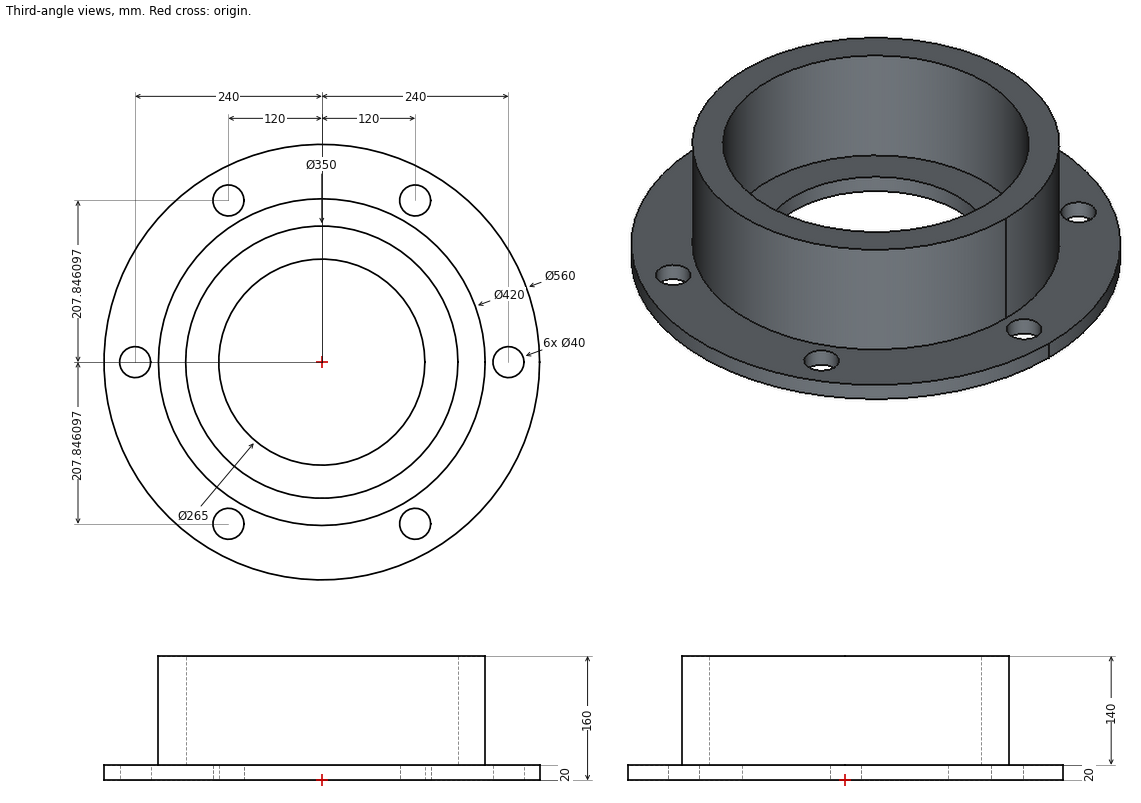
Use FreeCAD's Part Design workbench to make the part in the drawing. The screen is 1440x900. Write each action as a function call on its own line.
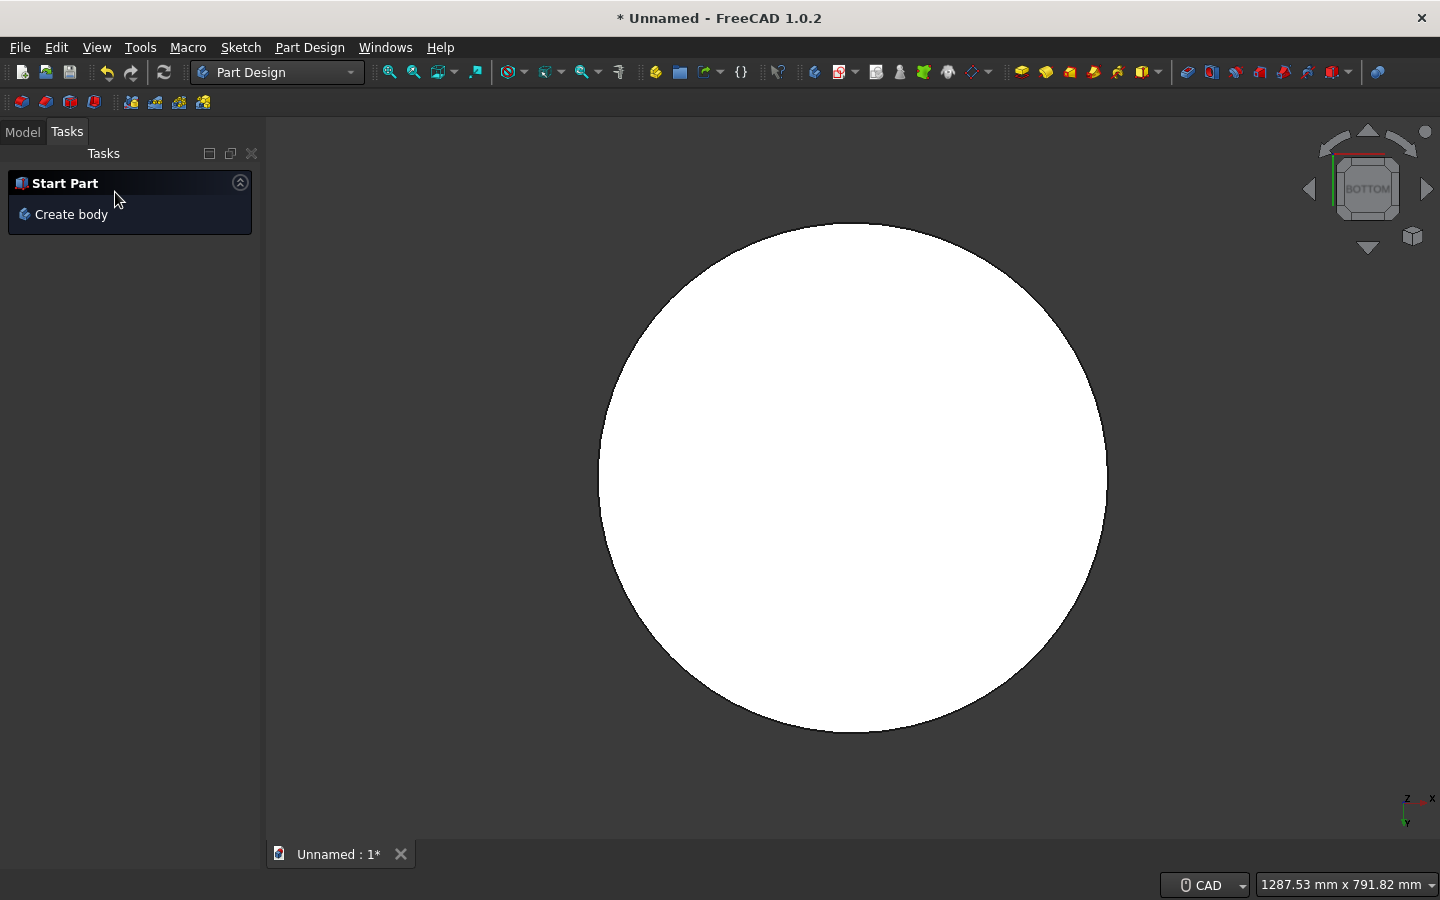
click(853, 477)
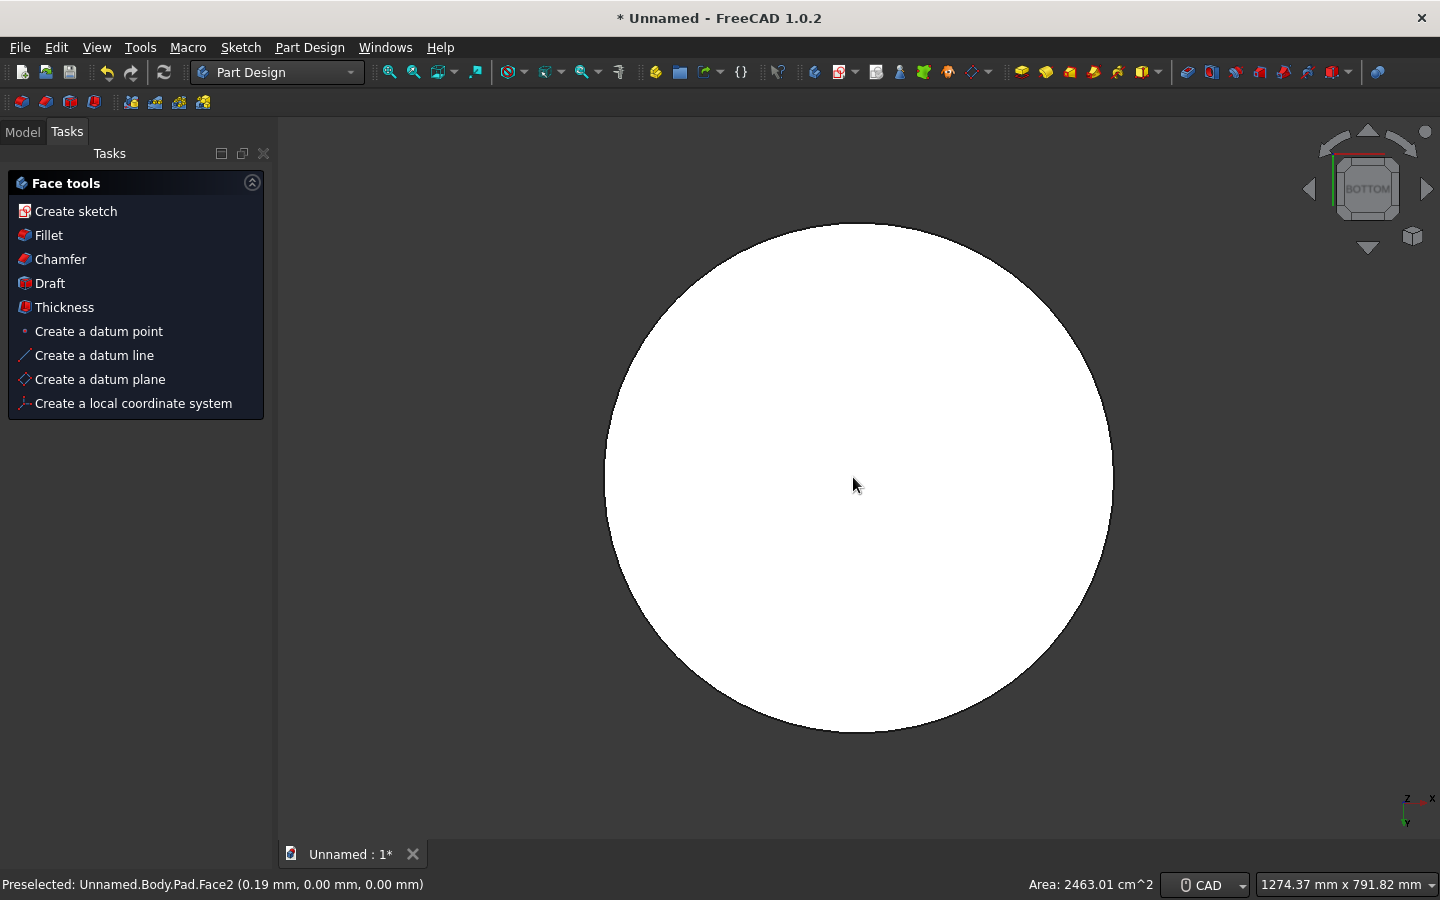
click(840, 72)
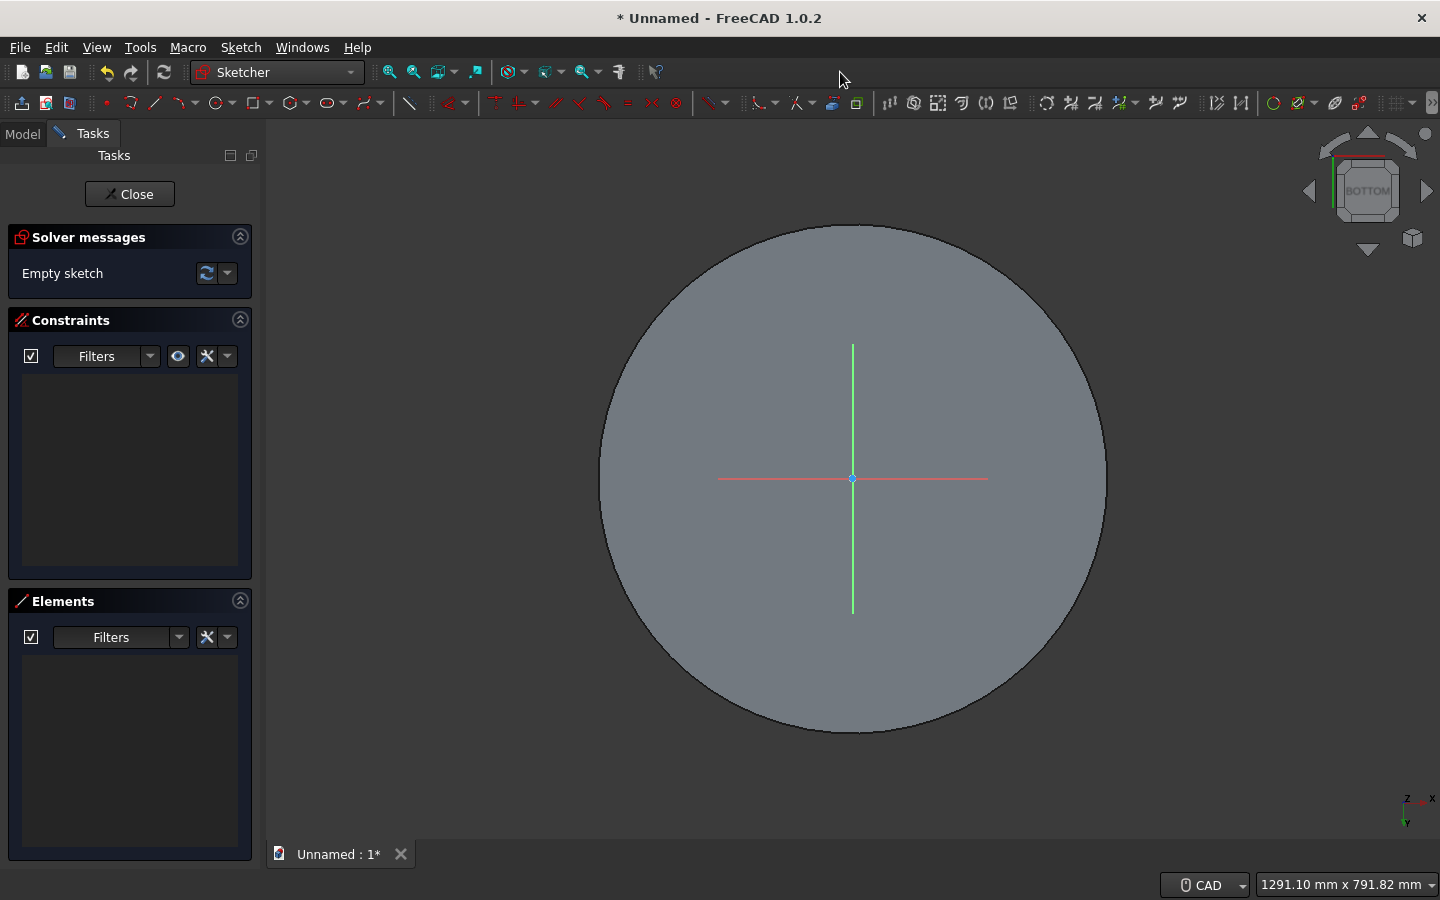
key(g)
key(c)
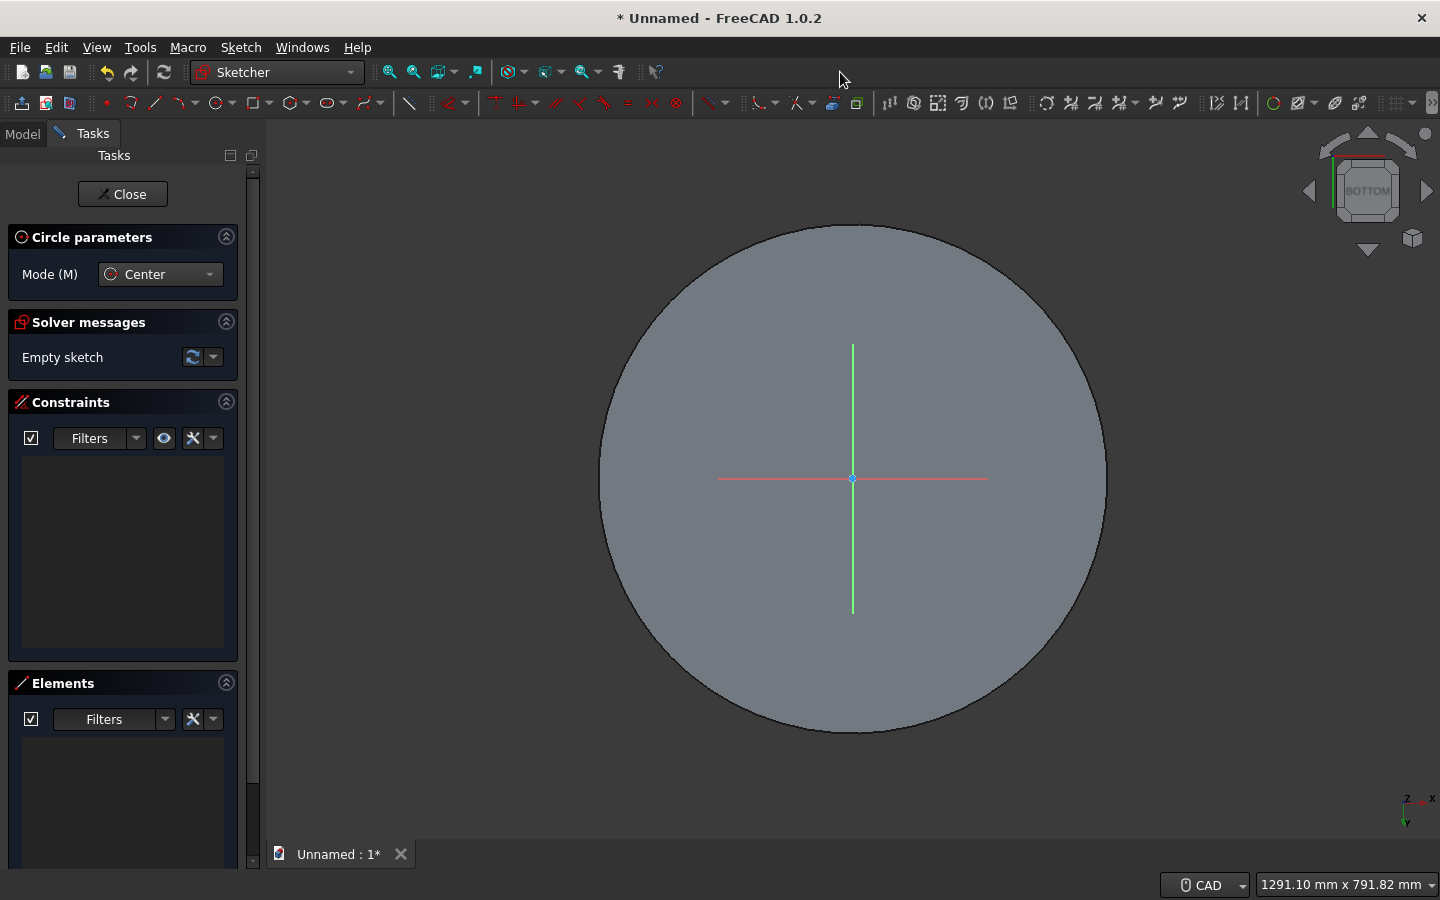
click(853, 479)
click(988, 344)
key(Escape)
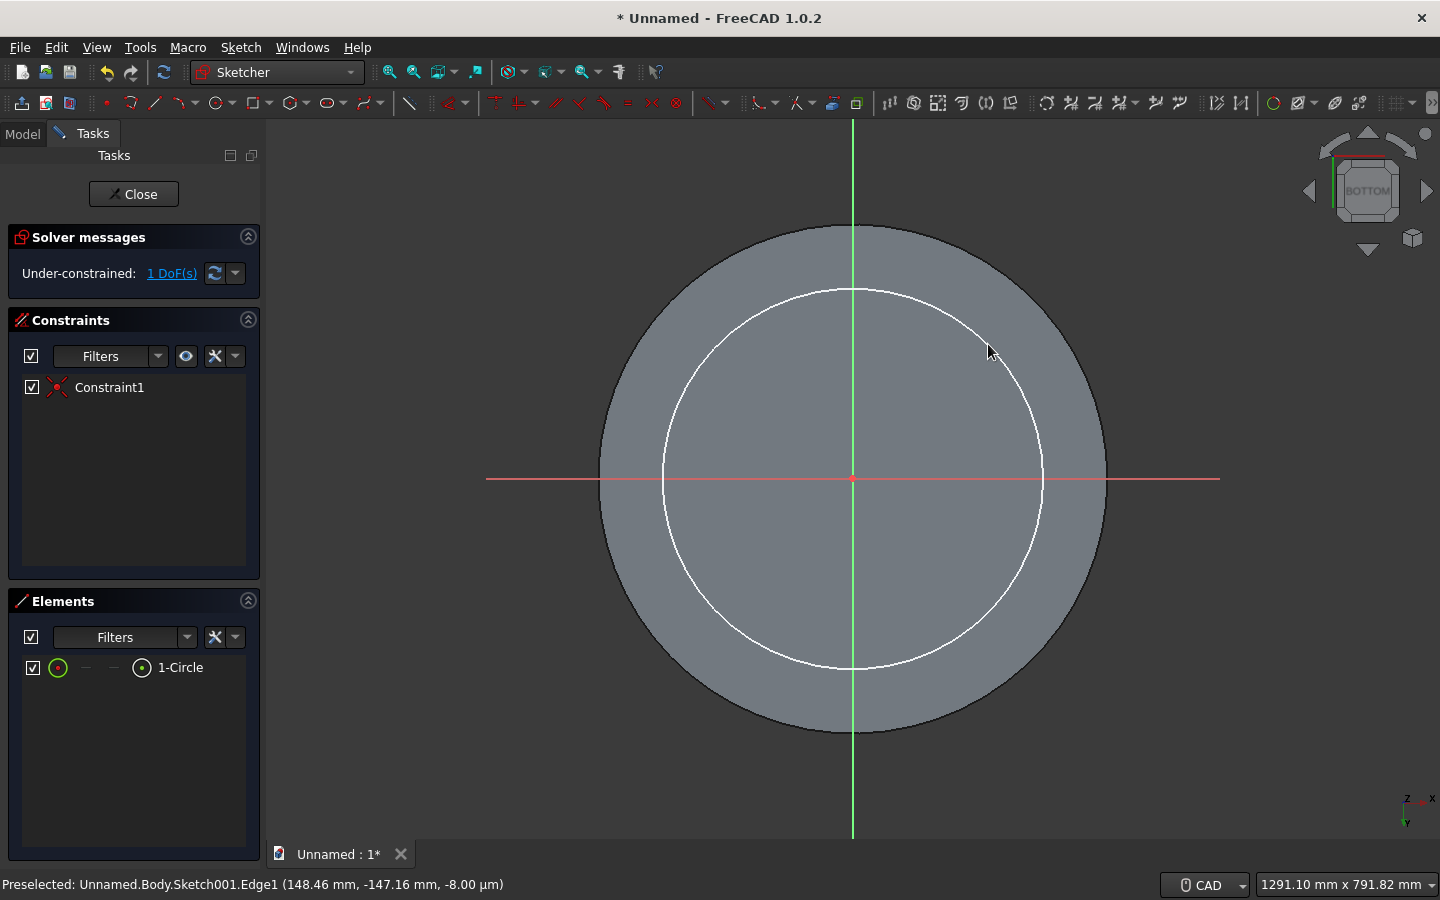
key(d)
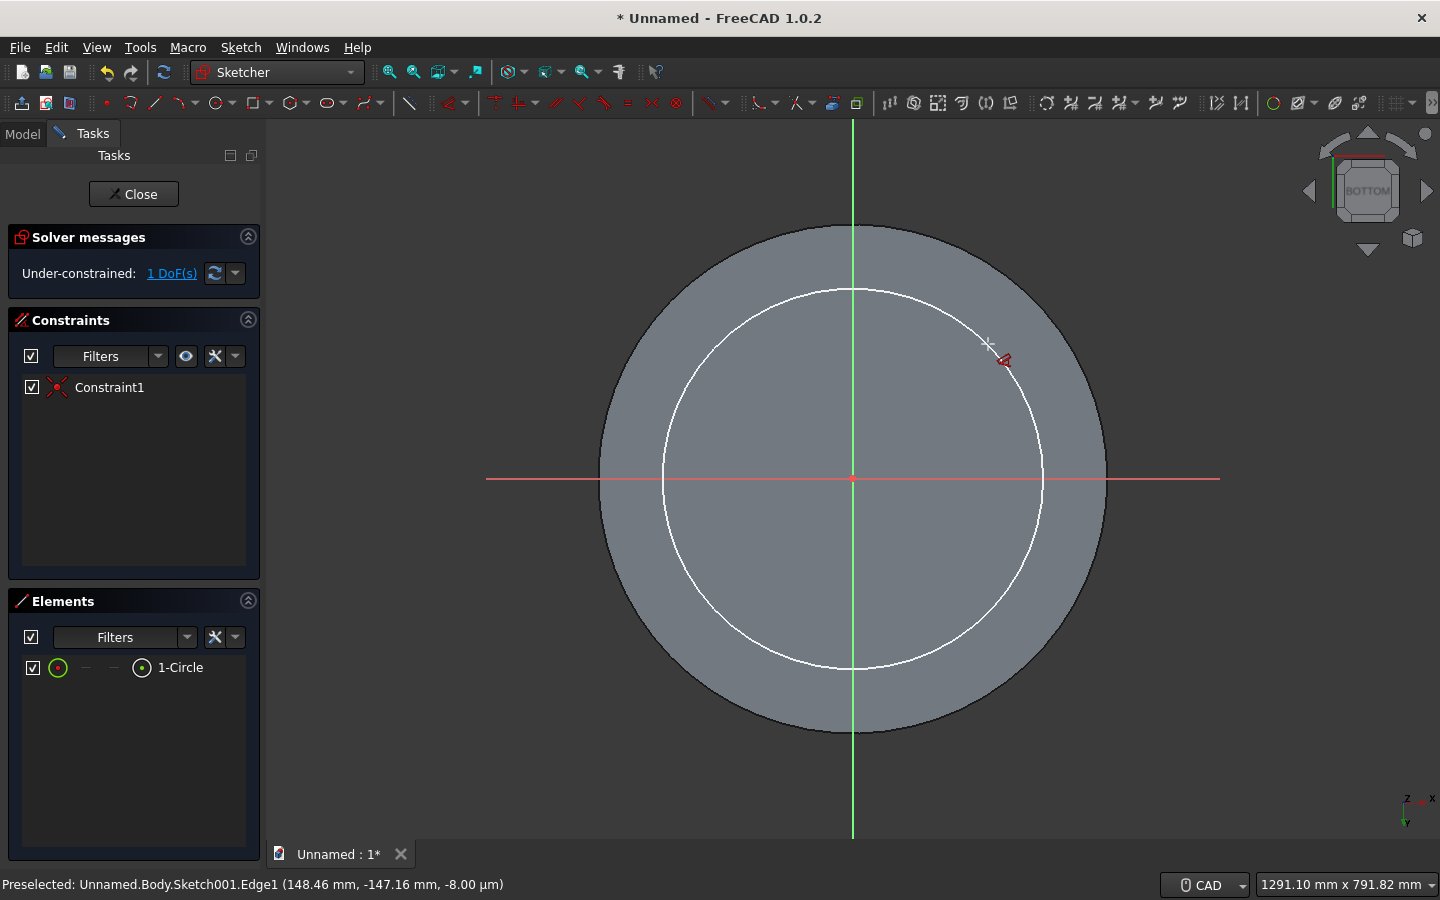
click(987, 344)
click(1010, 321)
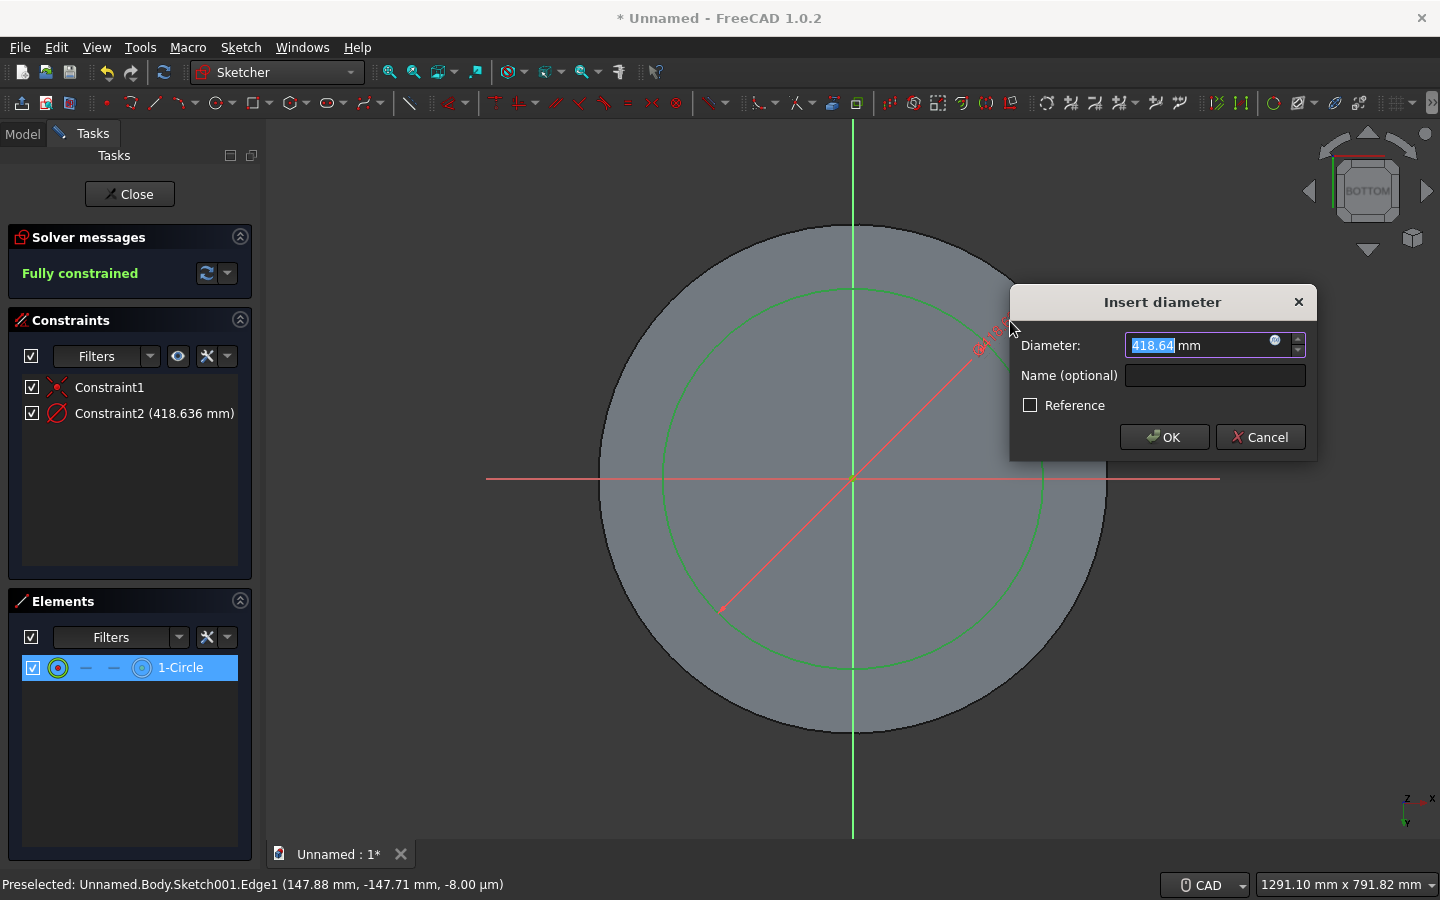
text(420)
key(Return)
key(Escape)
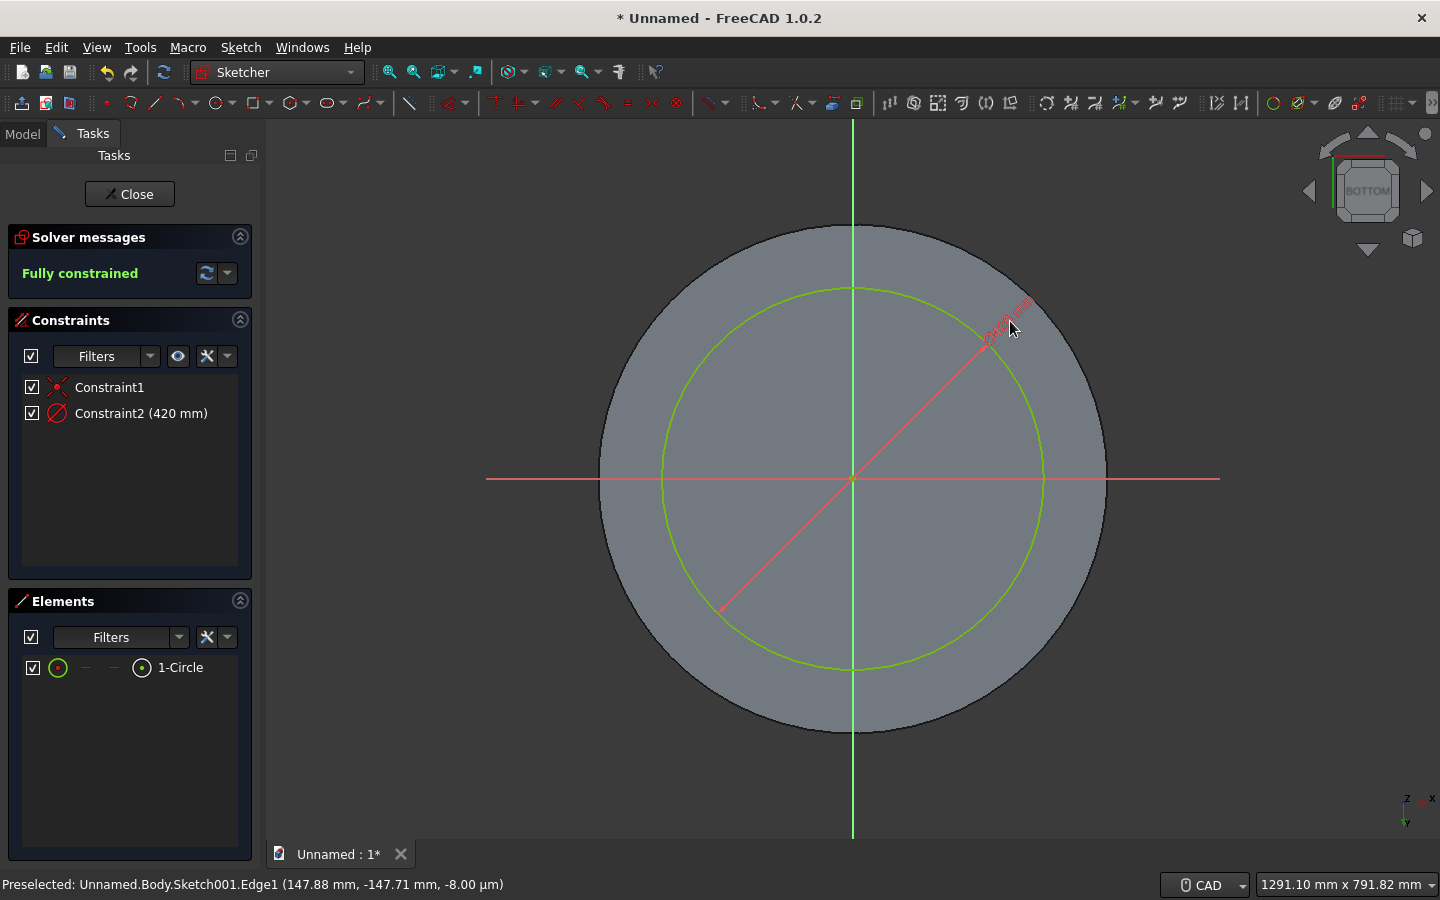
click(130, 194)